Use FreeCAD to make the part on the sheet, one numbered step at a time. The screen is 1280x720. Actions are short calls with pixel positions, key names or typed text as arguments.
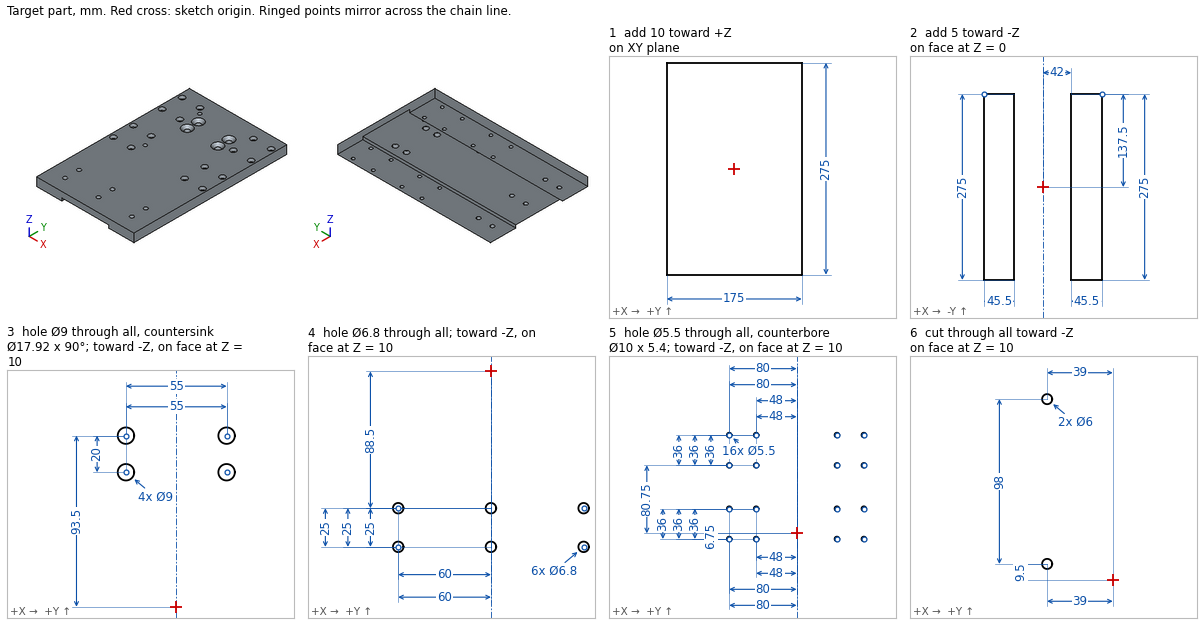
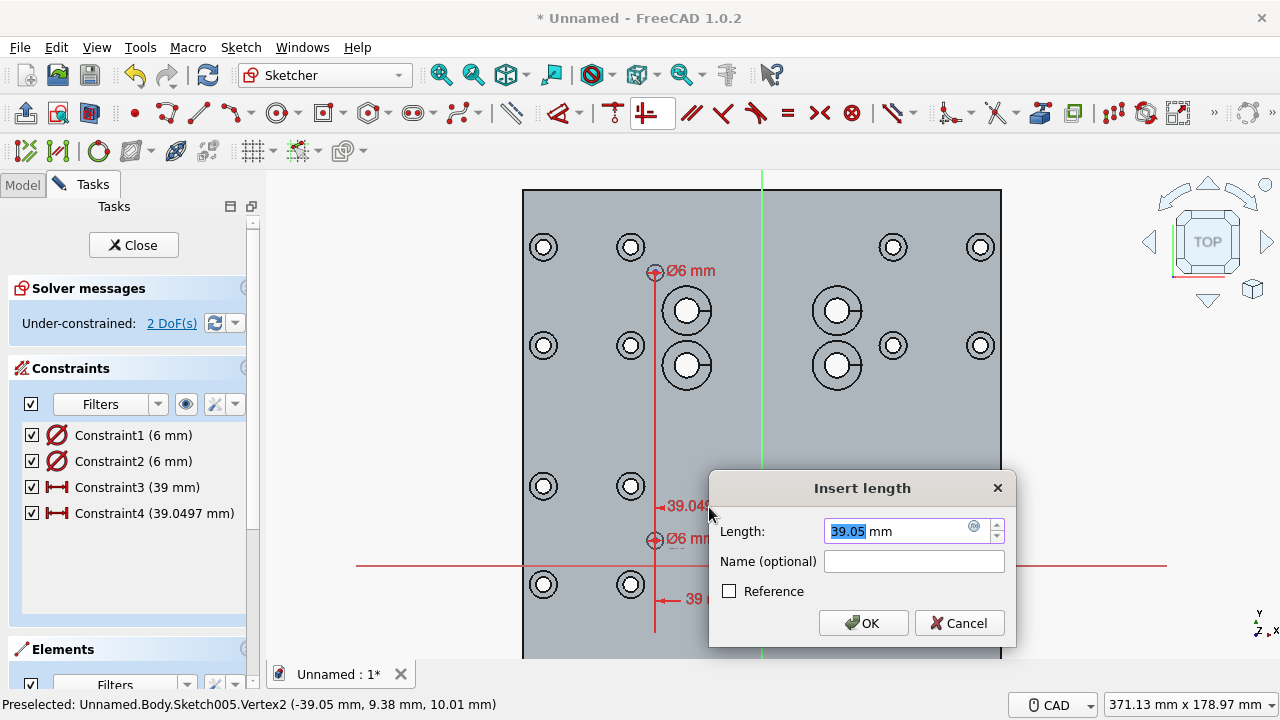
text(39)
key(Return)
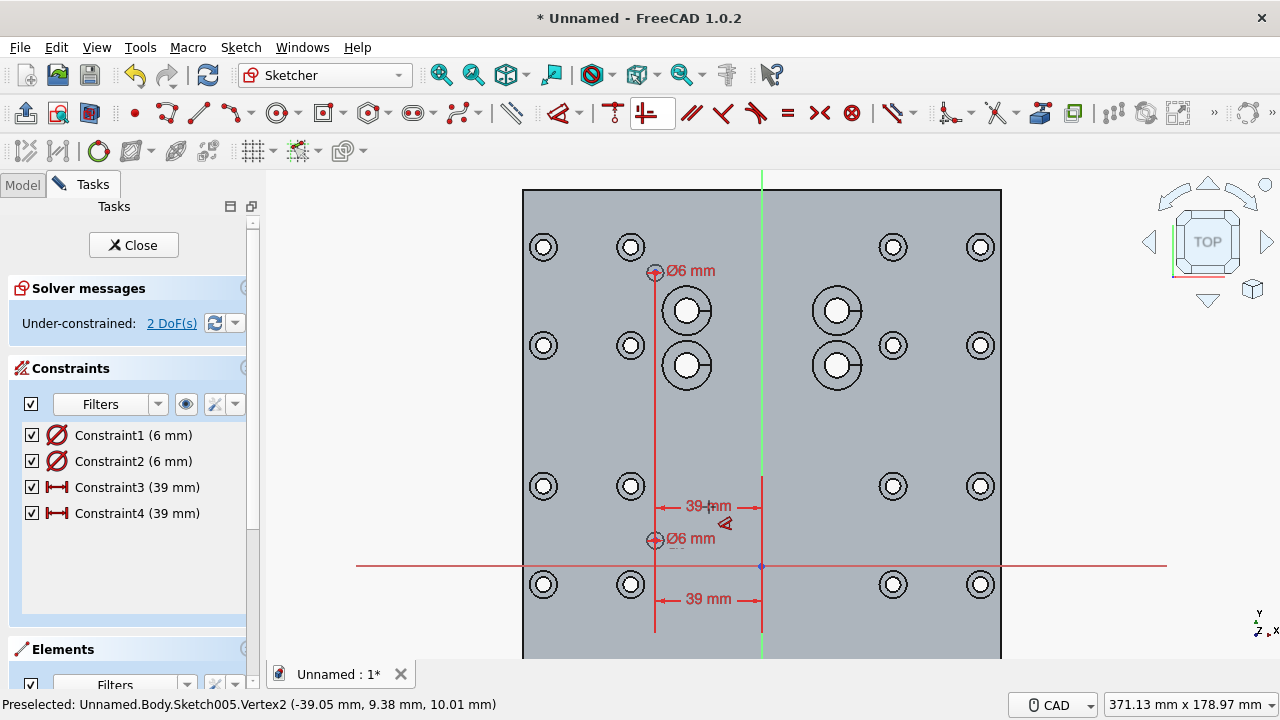
scroll(655, 541, up, 3)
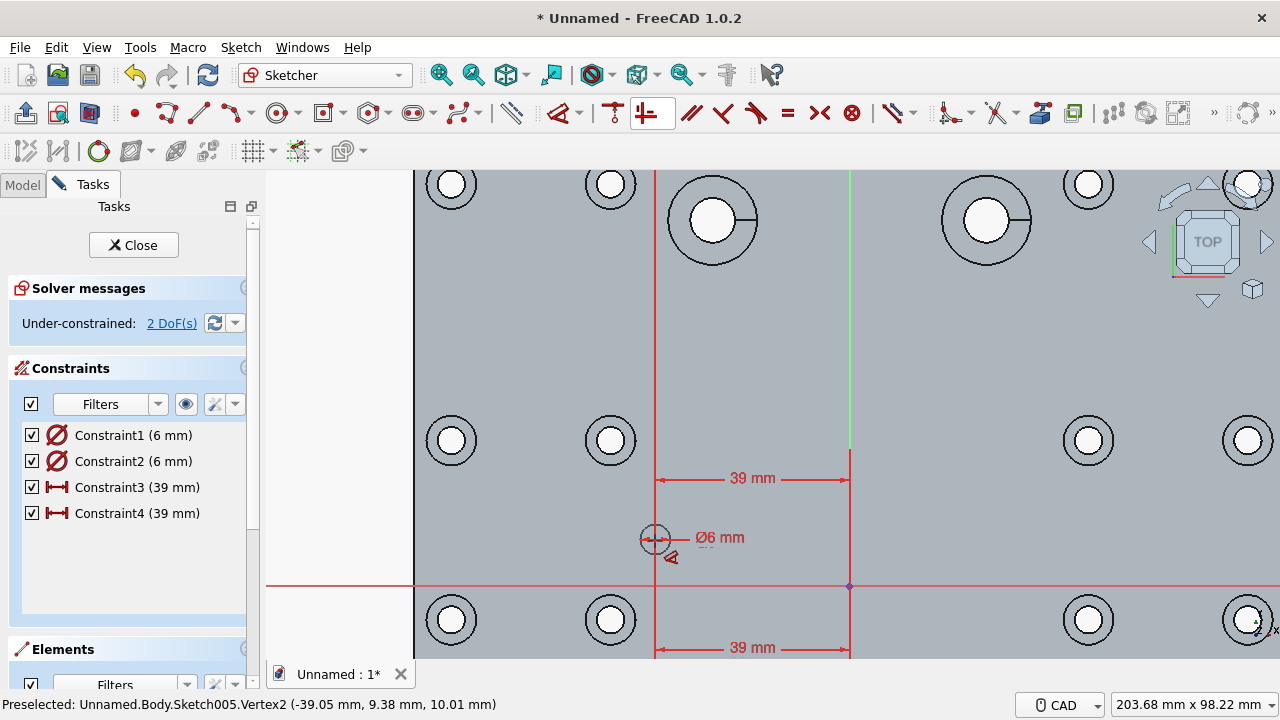
click(655, 540)
click(884, 563)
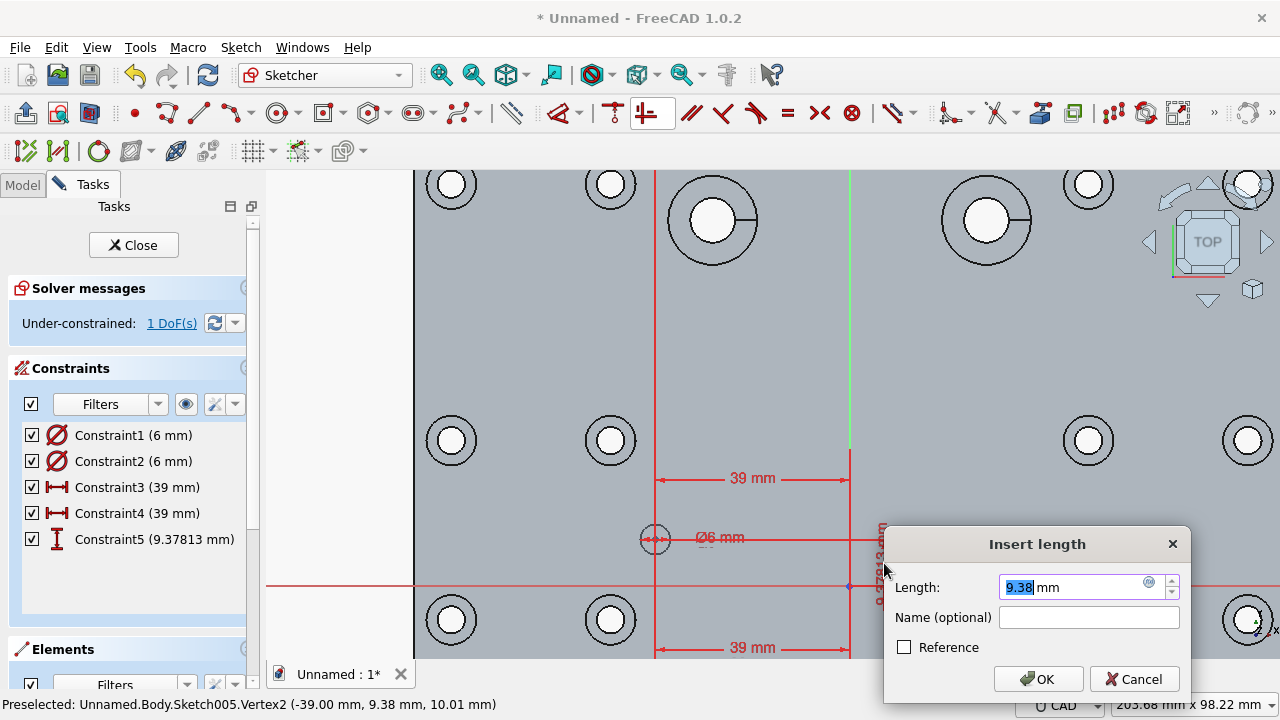
text(9.5)
key(Return)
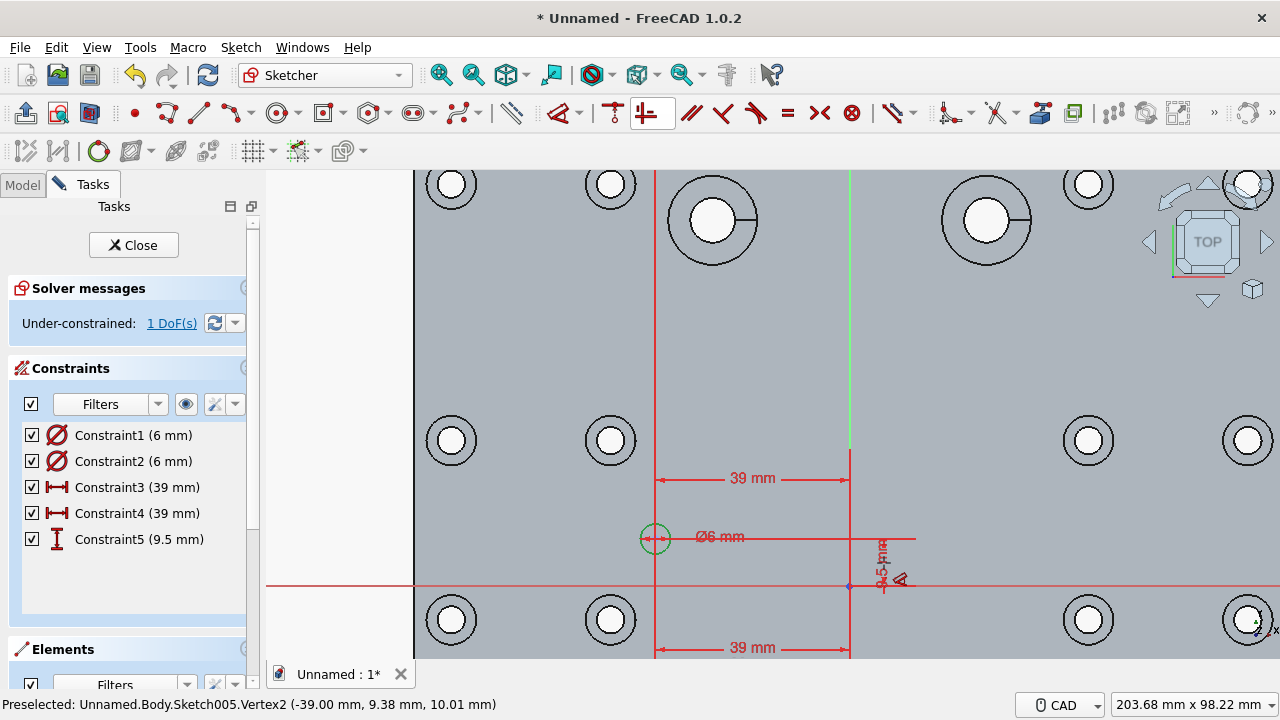
scroll(655, 540, down, 3)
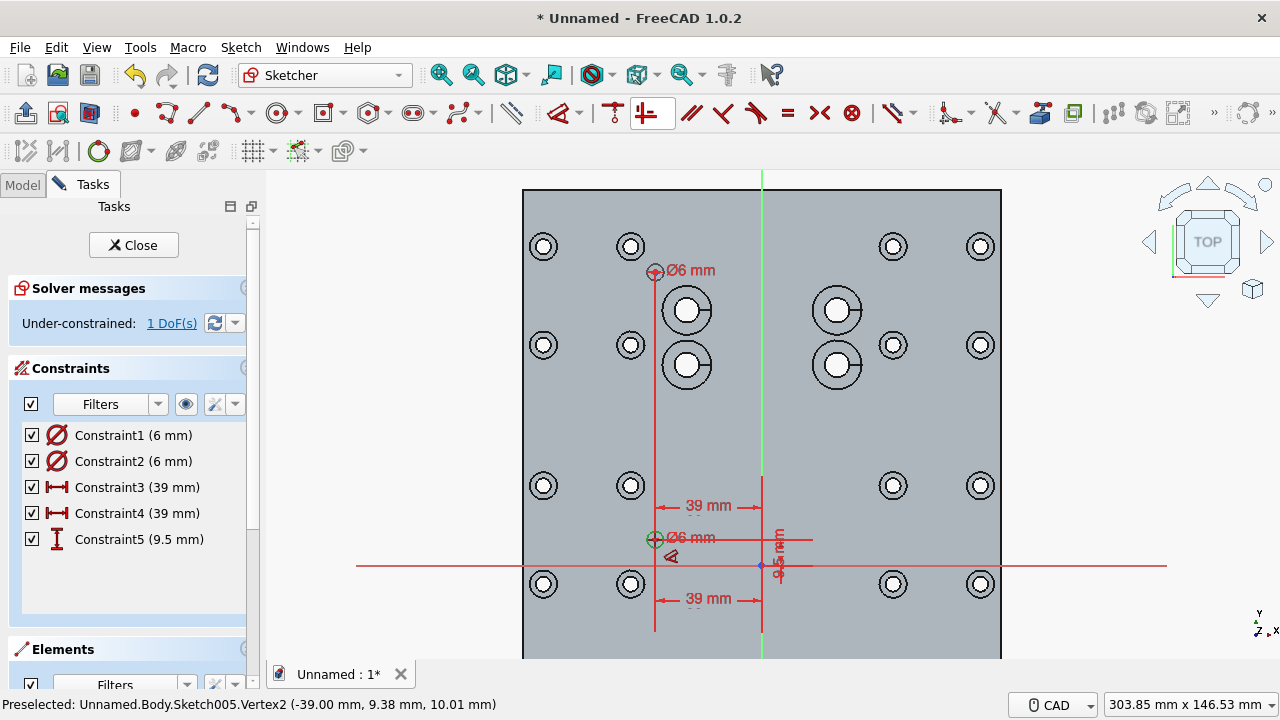
click(655, 272)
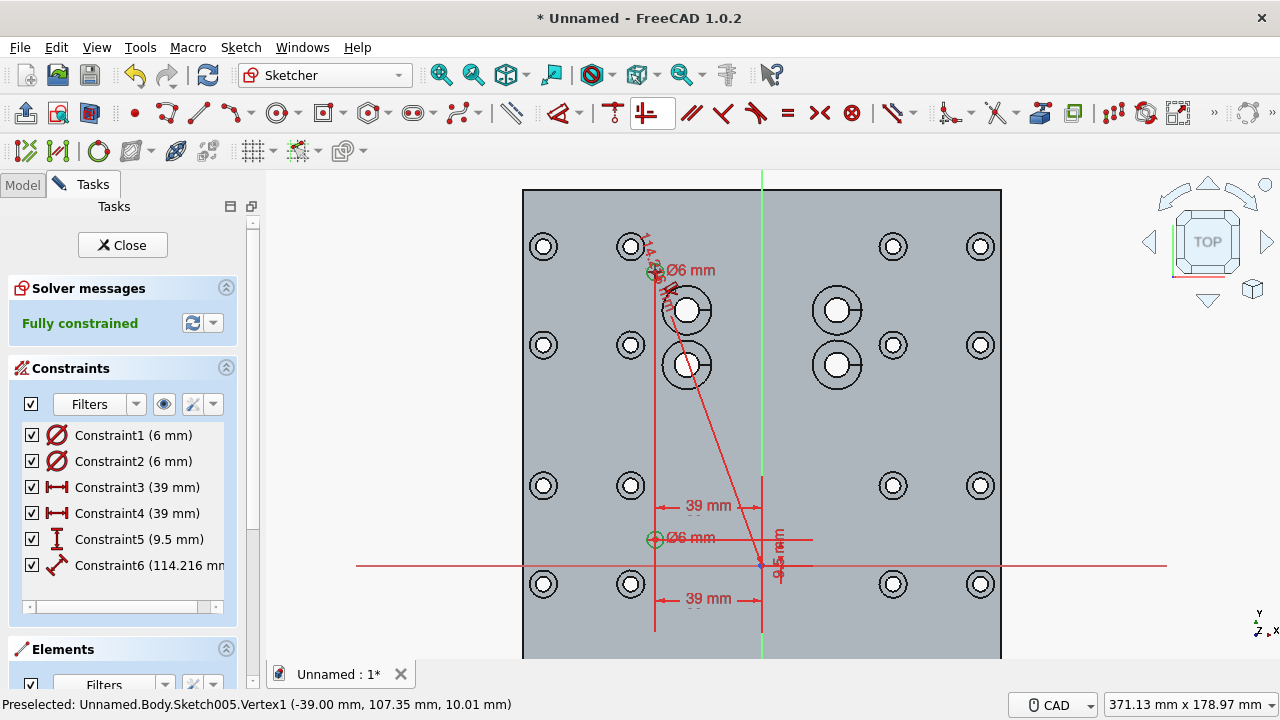
click(655, 540)
click(621, 406)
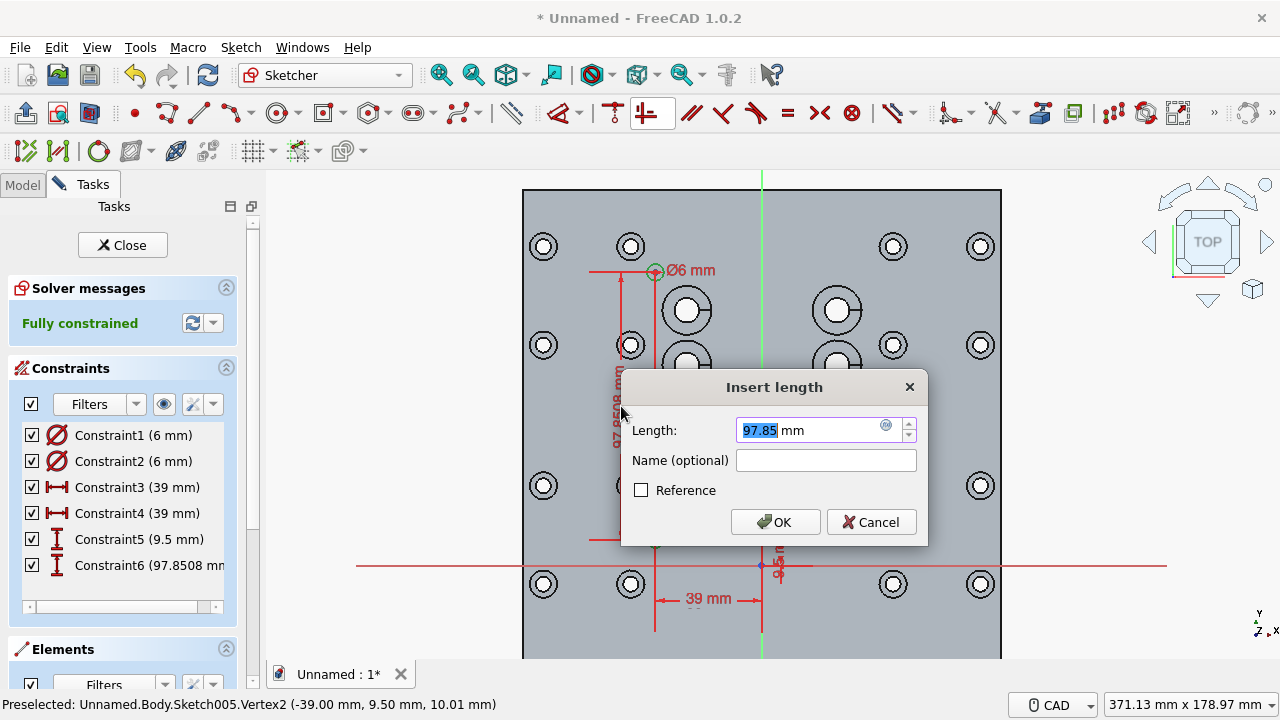
text(98)
key(Return)
key(Escape)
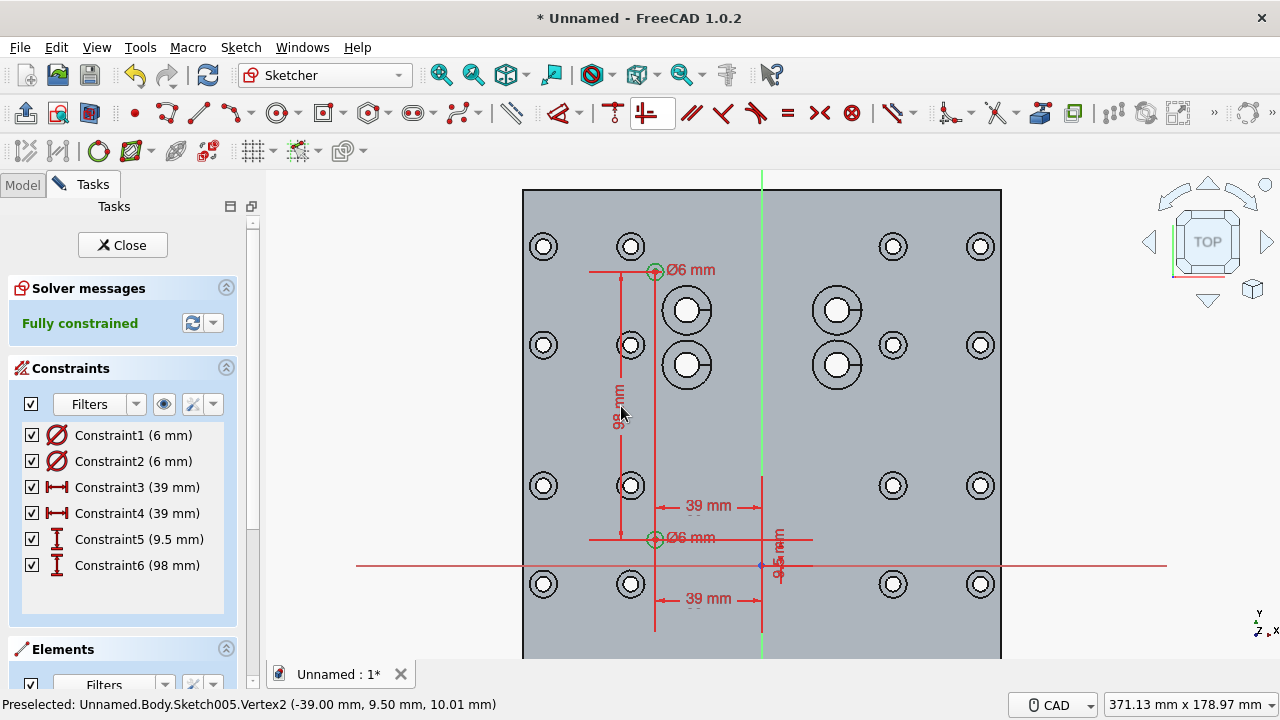
click(123, 245)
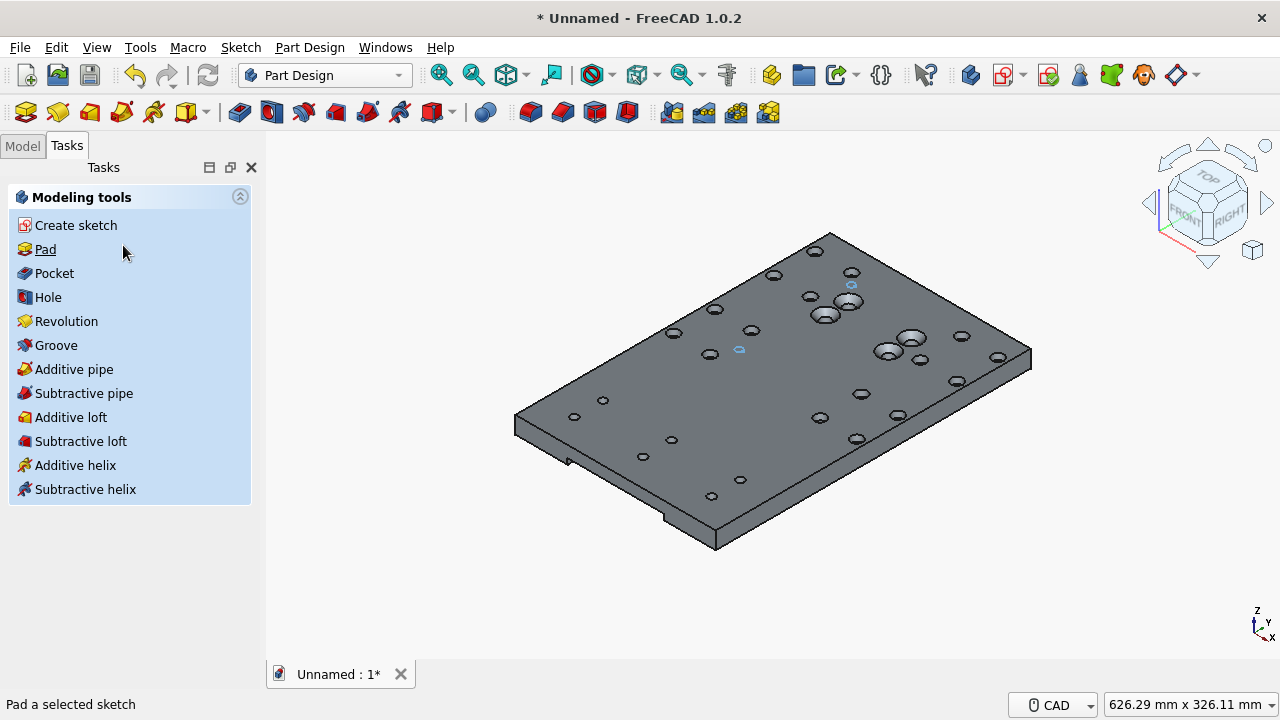
click(240, 112)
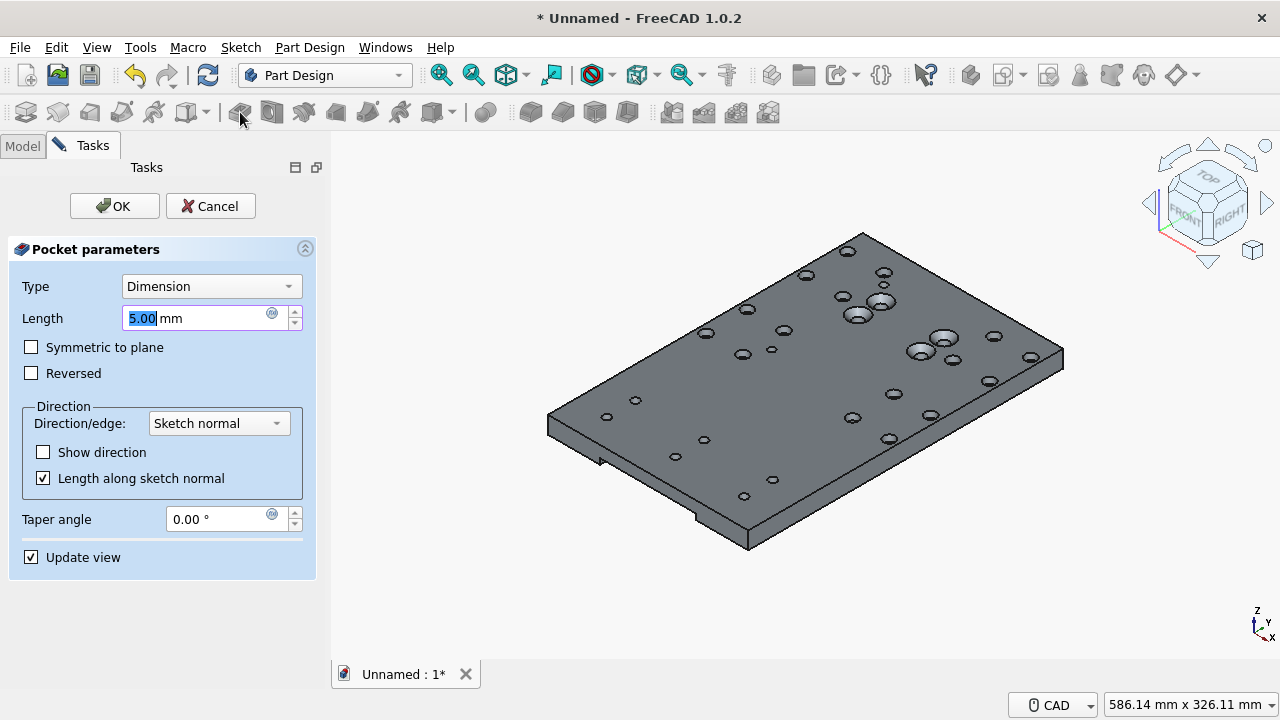
click(212, 286)